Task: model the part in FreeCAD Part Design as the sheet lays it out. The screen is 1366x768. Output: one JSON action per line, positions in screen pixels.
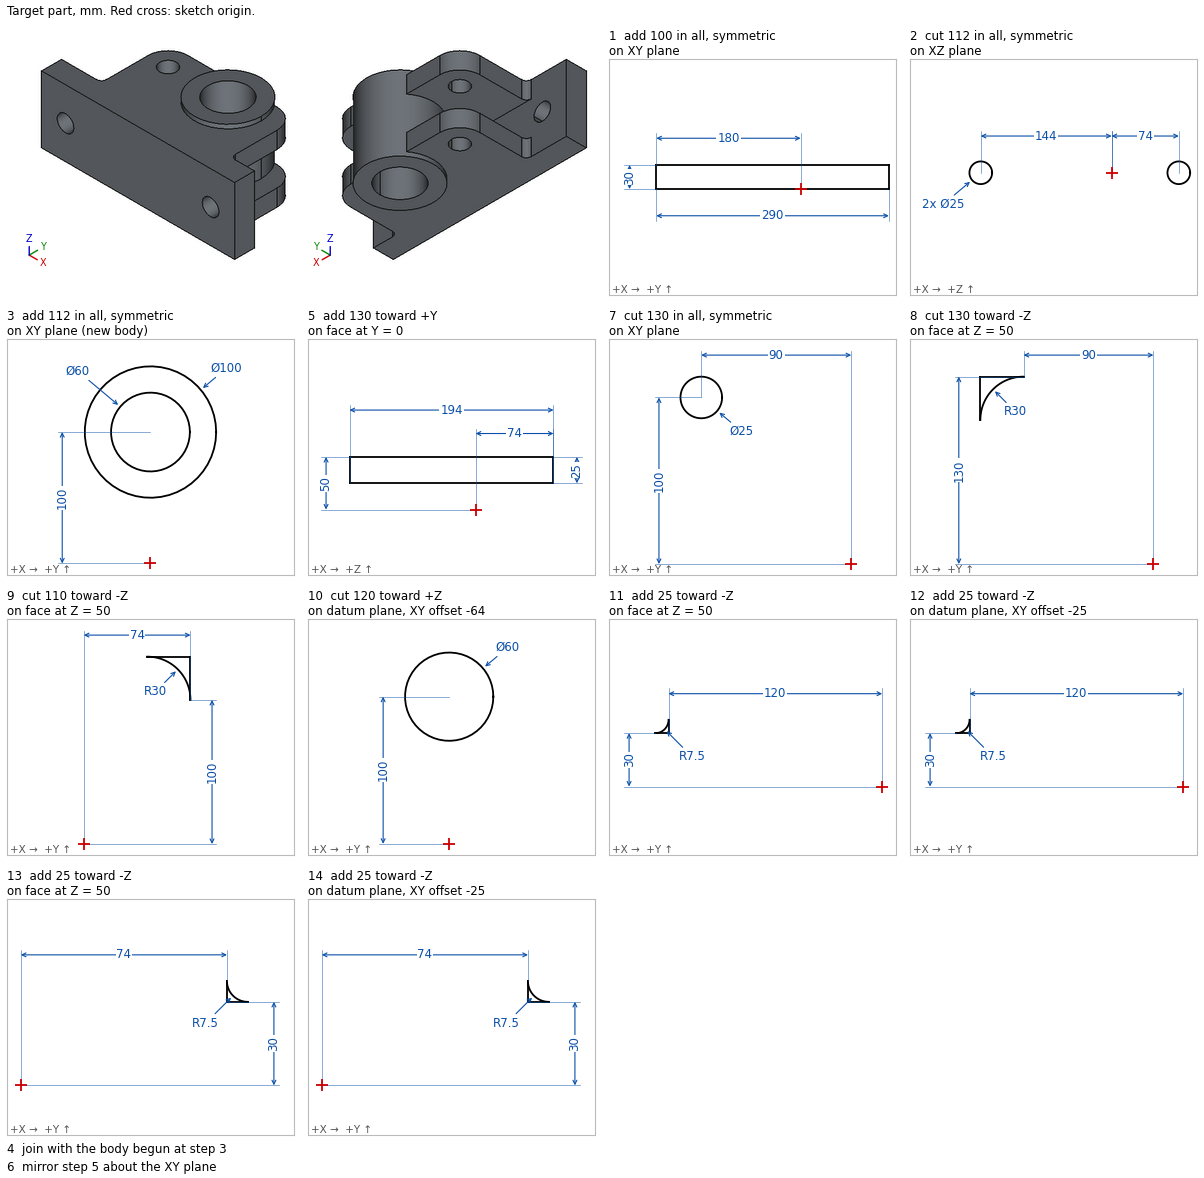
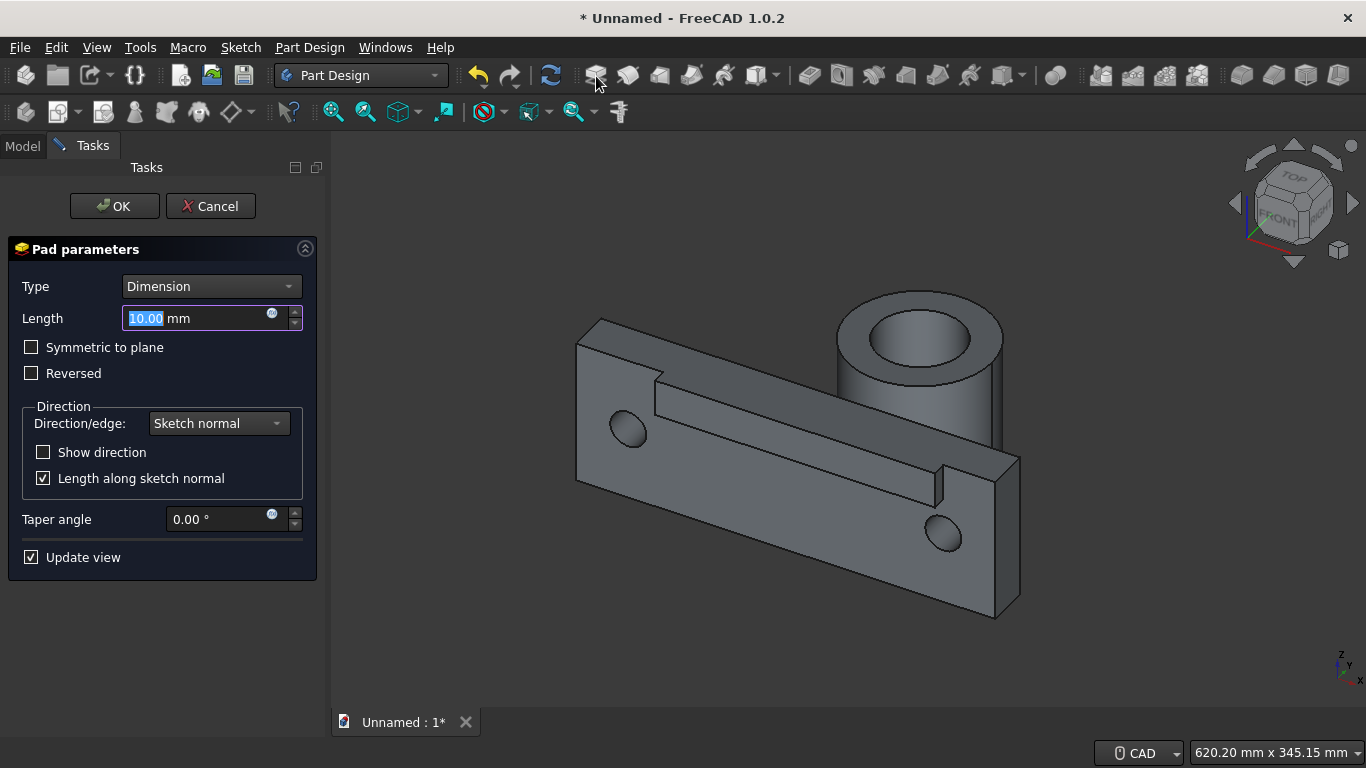
{"action": "type", "text": "130"}
{"action": "key", "text": "Tab"}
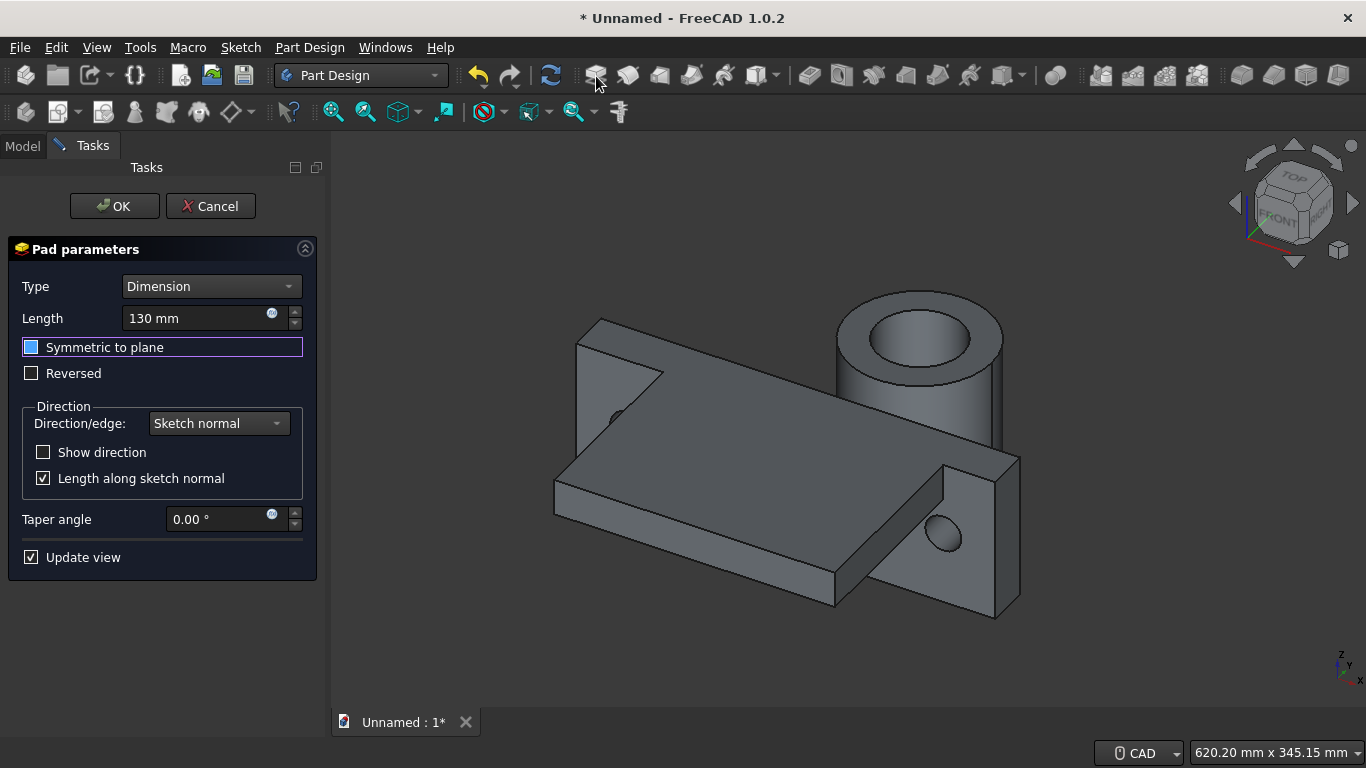
{"action": "left_click", "coordinate": [30, 373]}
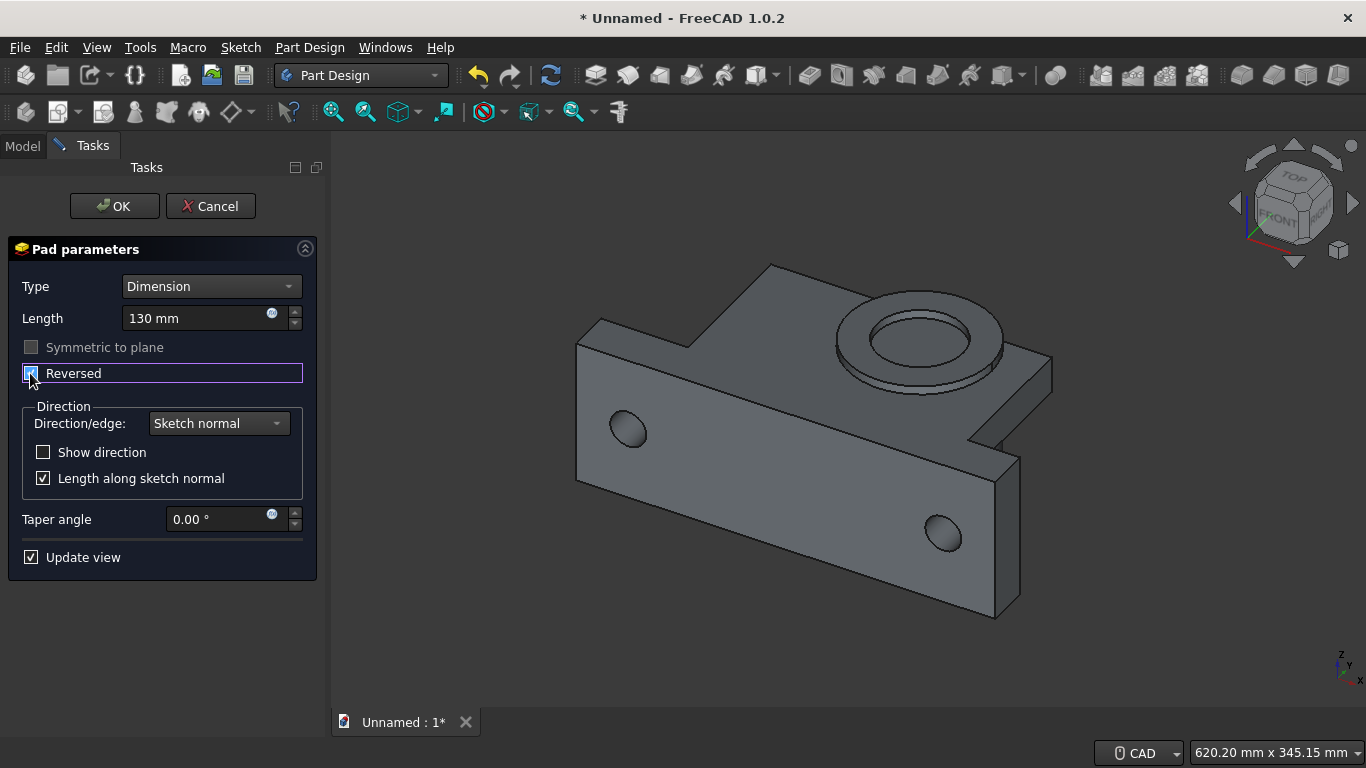
{"action": "left_click", "coordinate": [115, 206]}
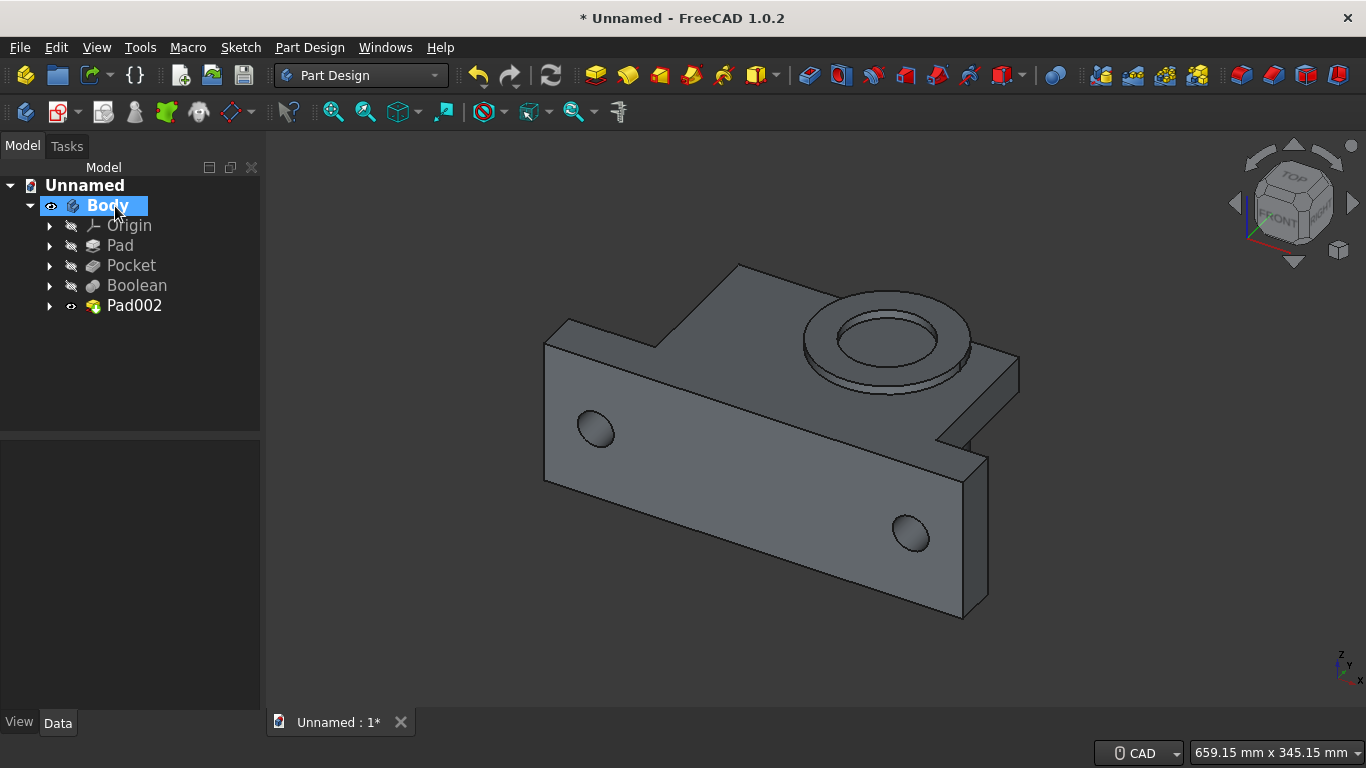
{"action": "left_click", "coordinate": [116, 306]}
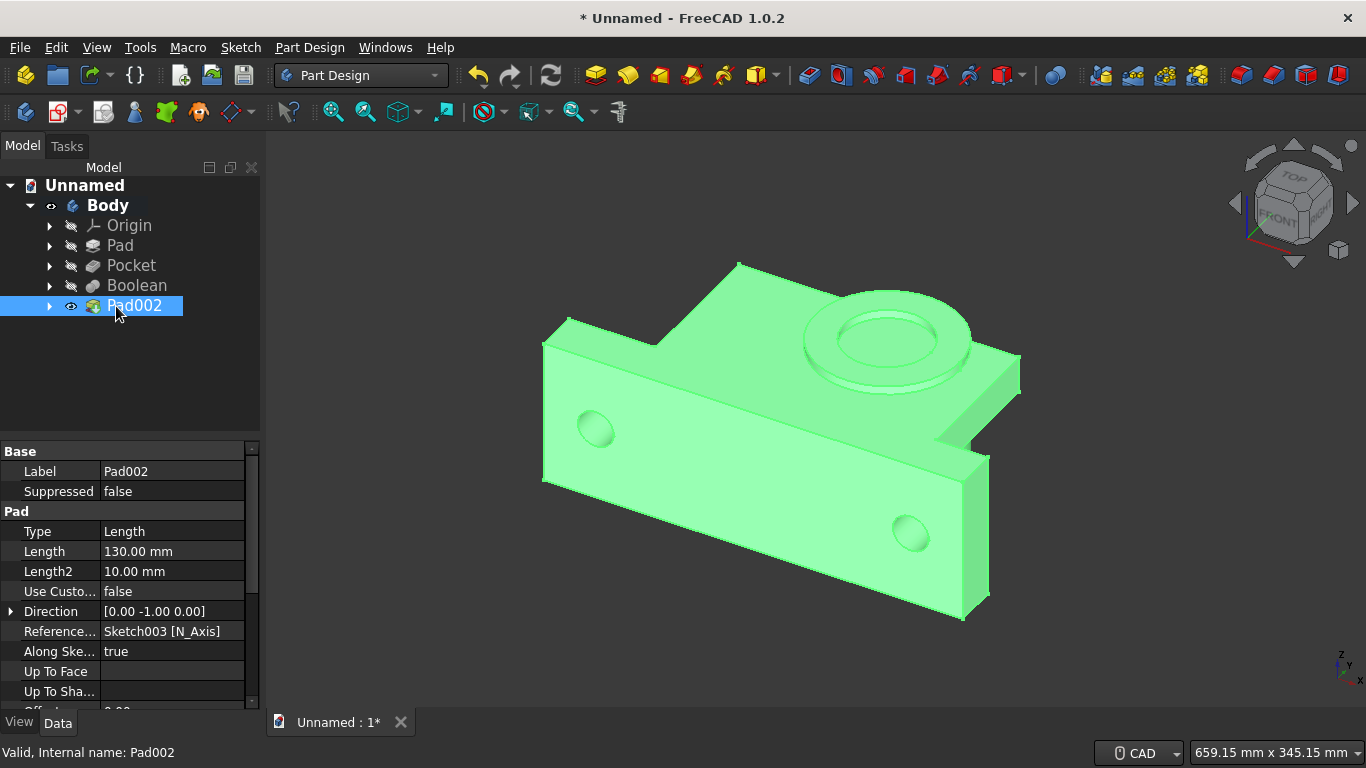
{"action": "left_click", "coordinate": [1102, 76]}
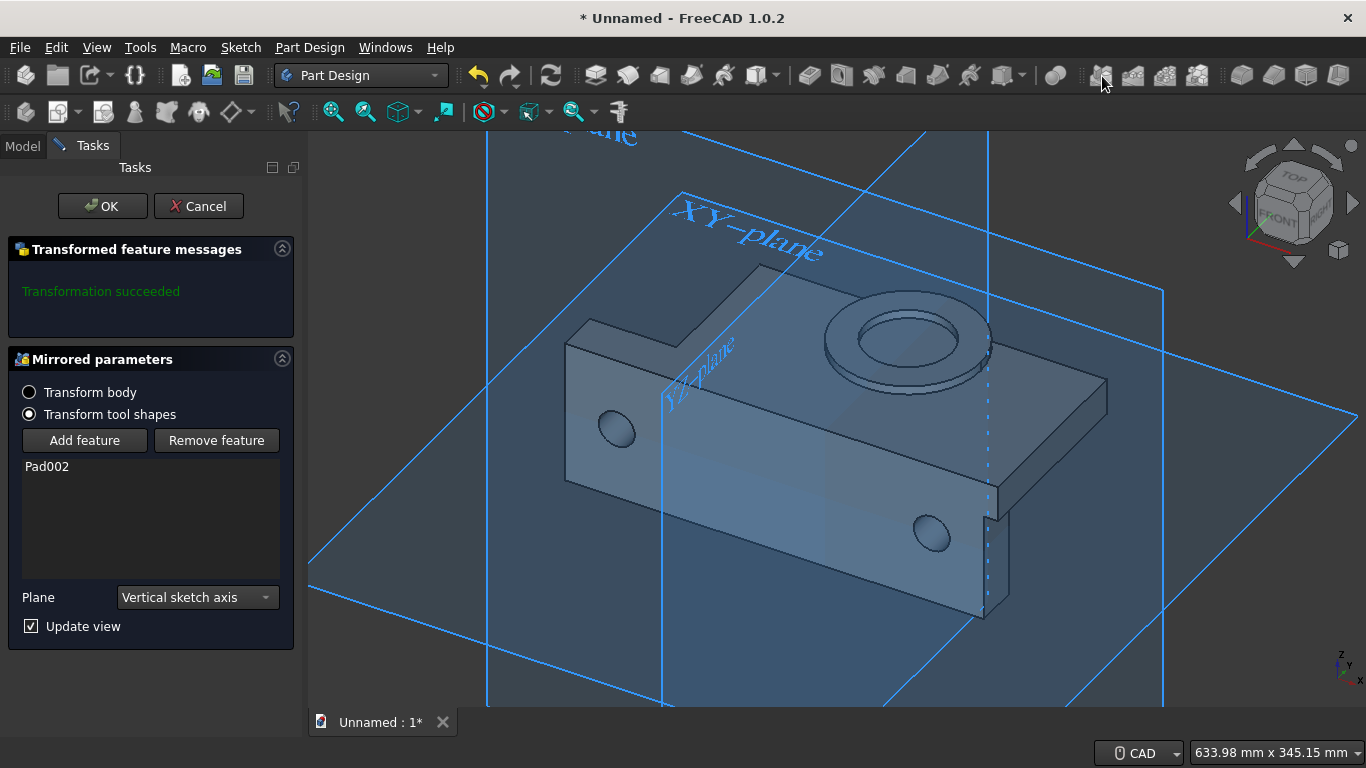
{"action": "left_click", "coordinate": [198, 598]}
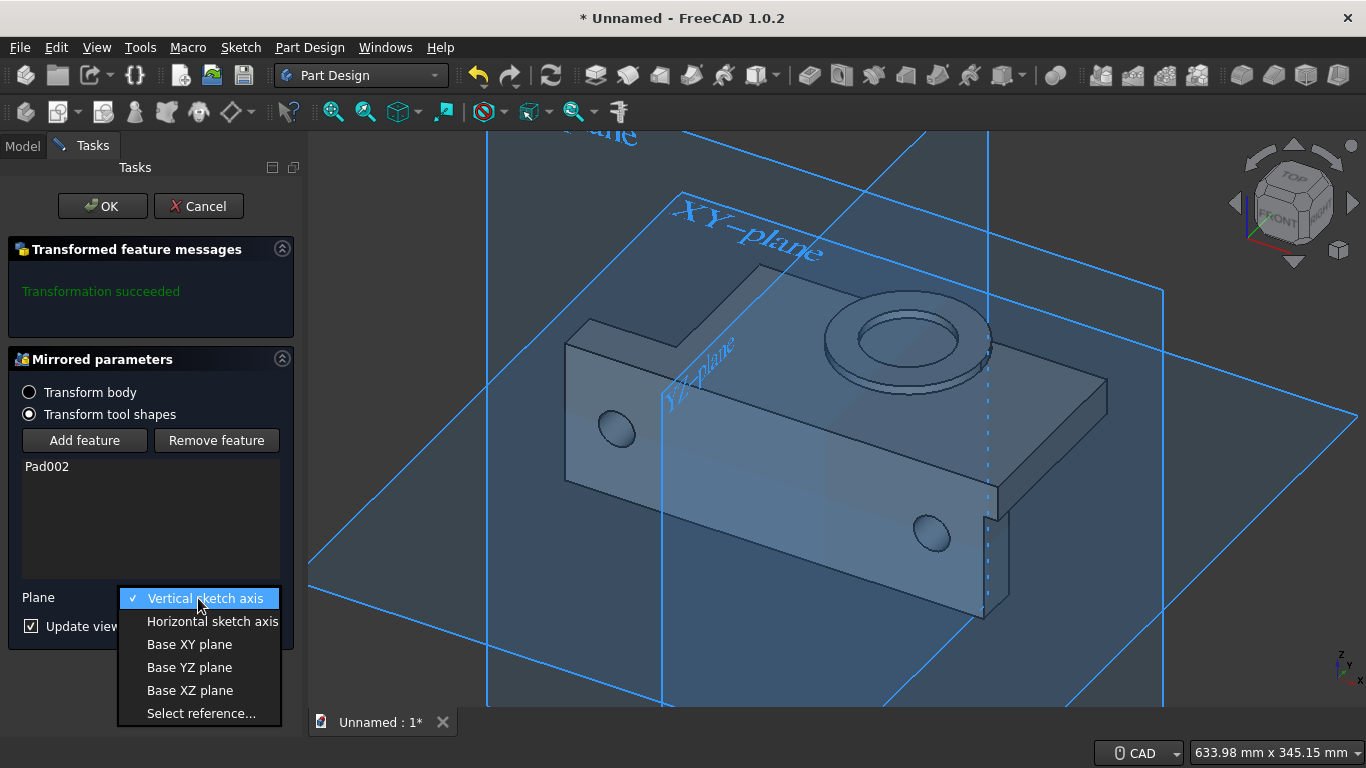
{"action": "left_click", "coordinate": [198, 644]}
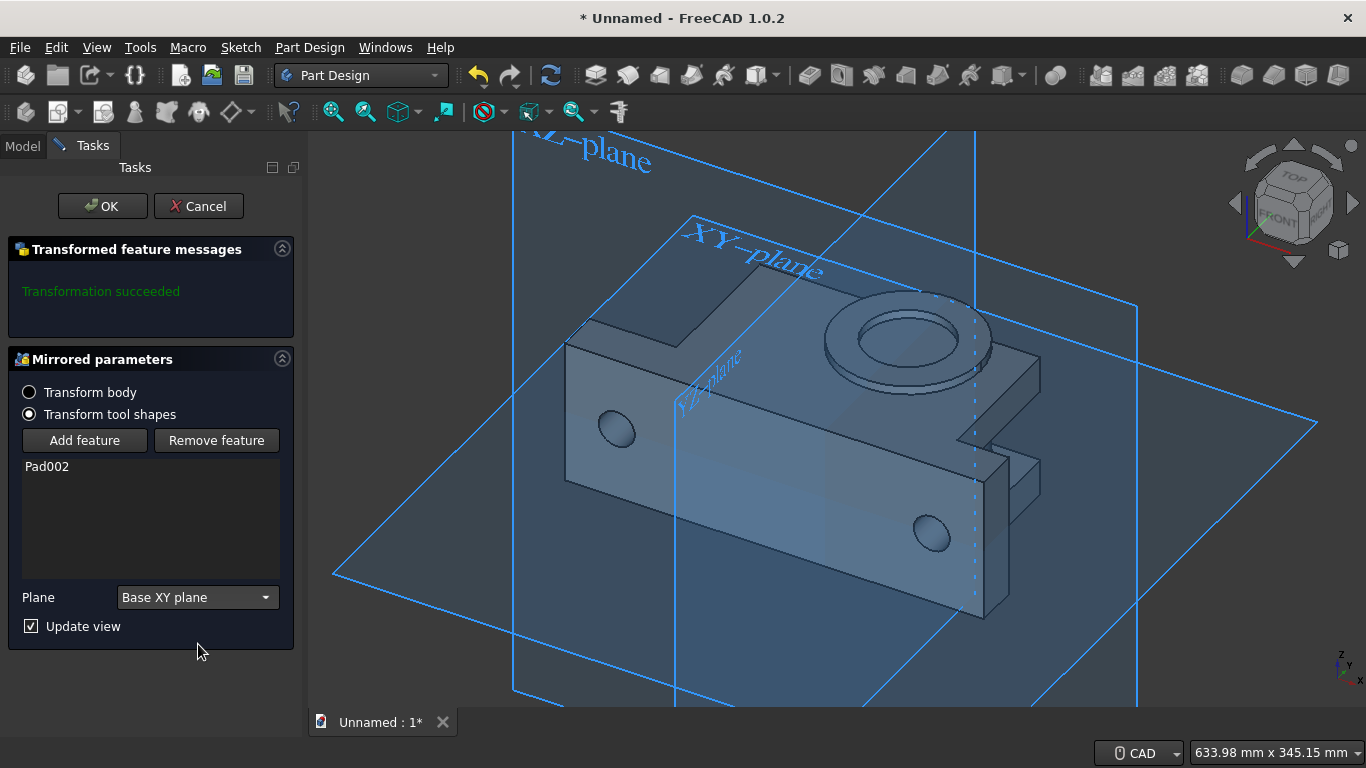
{"action": "left_click", "coordinate": [103, 206]}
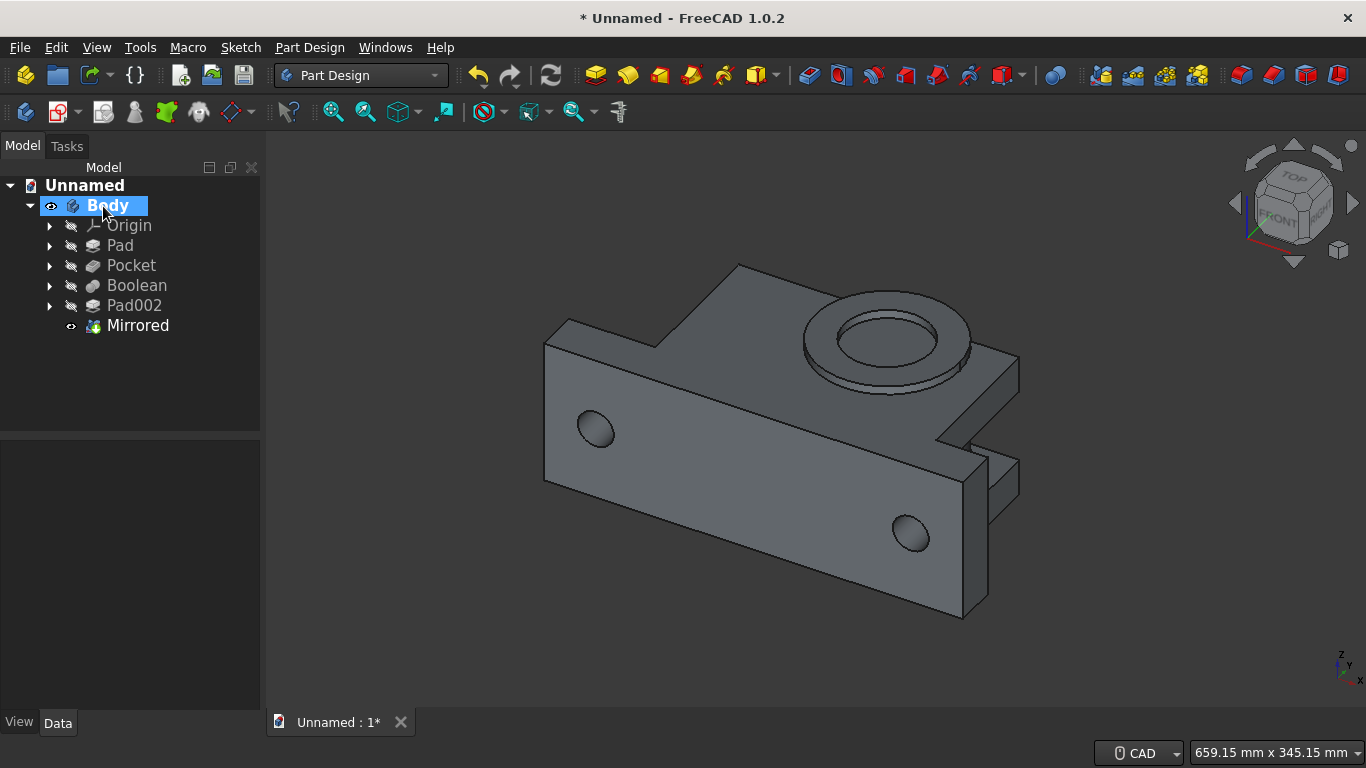
{"action": "left_click", "coordinate": [58, 112]}